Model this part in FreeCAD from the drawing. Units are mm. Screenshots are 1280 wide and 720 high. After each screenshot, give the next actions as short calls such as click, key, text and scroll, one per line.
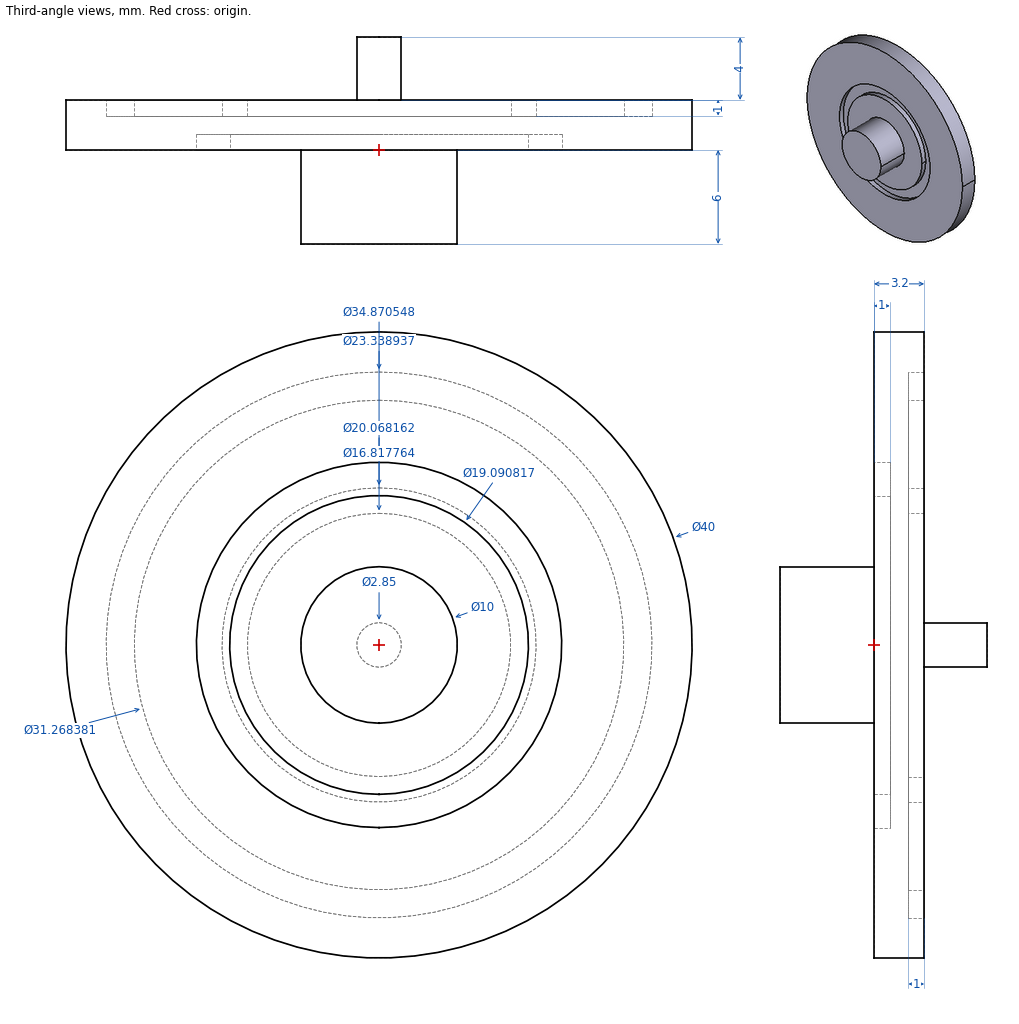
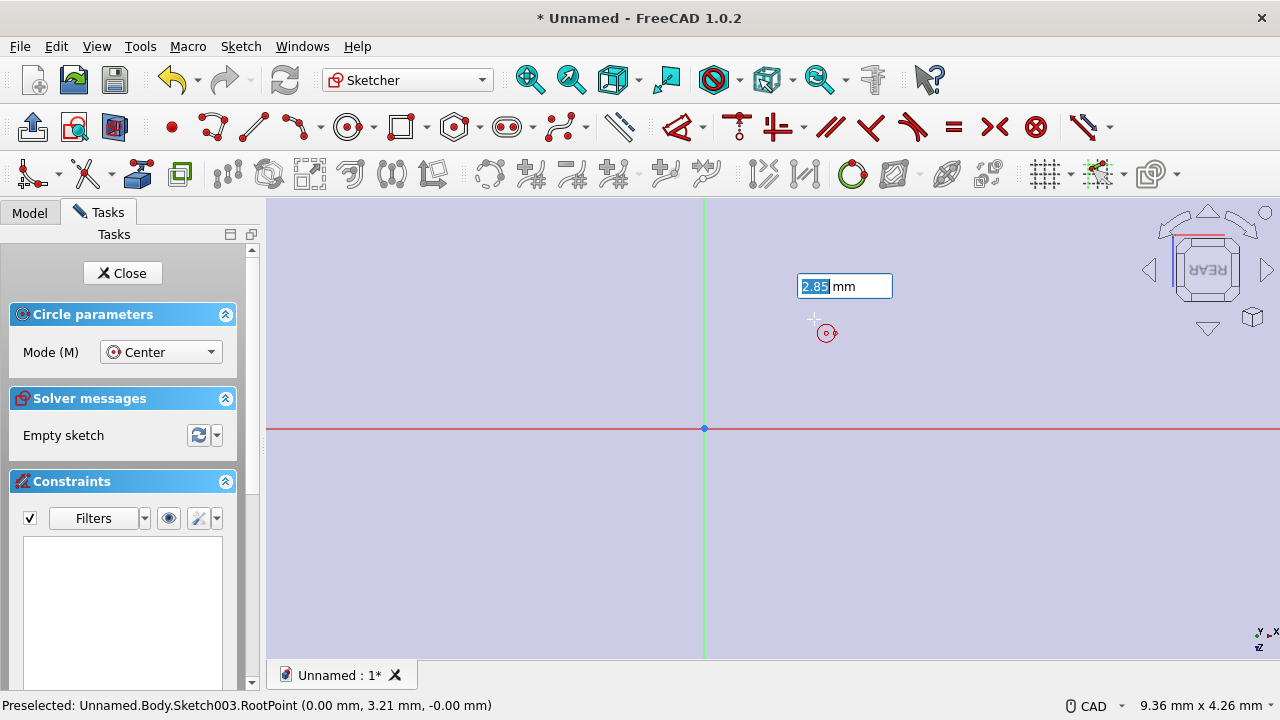
text(2.85)
key(Return)
key(Escape)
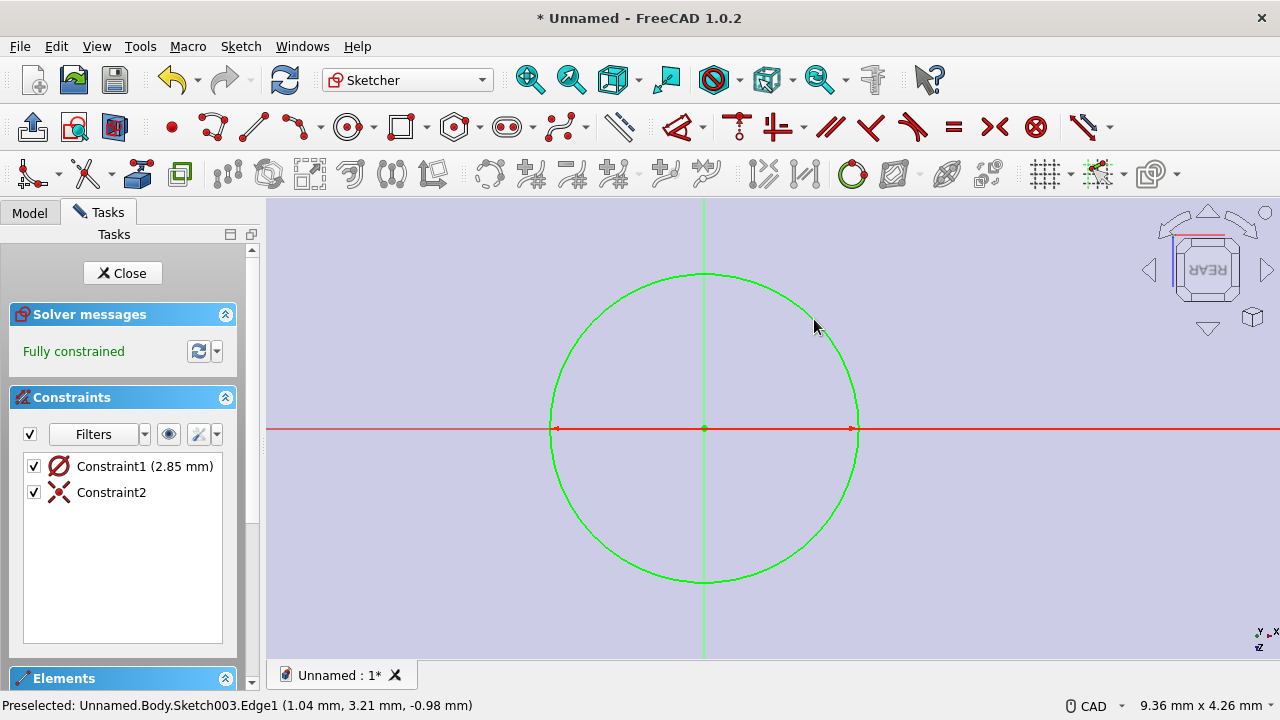
click(123, 273)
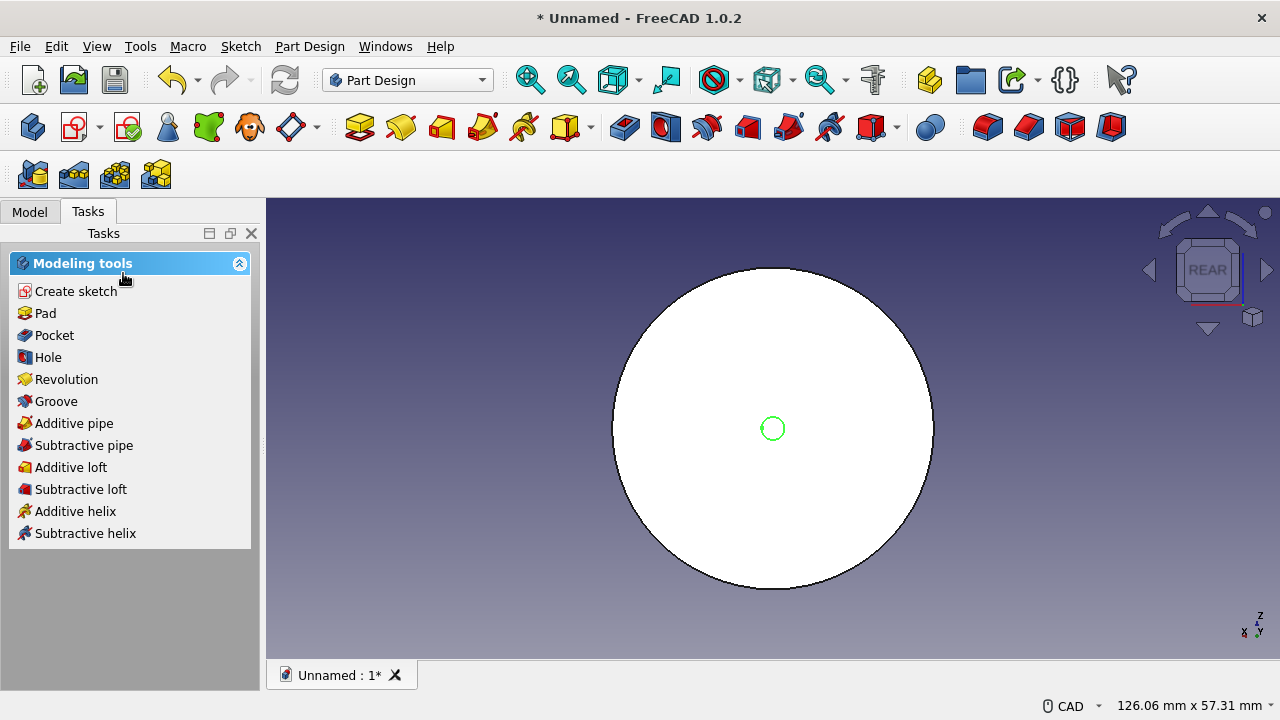
click(360, 128)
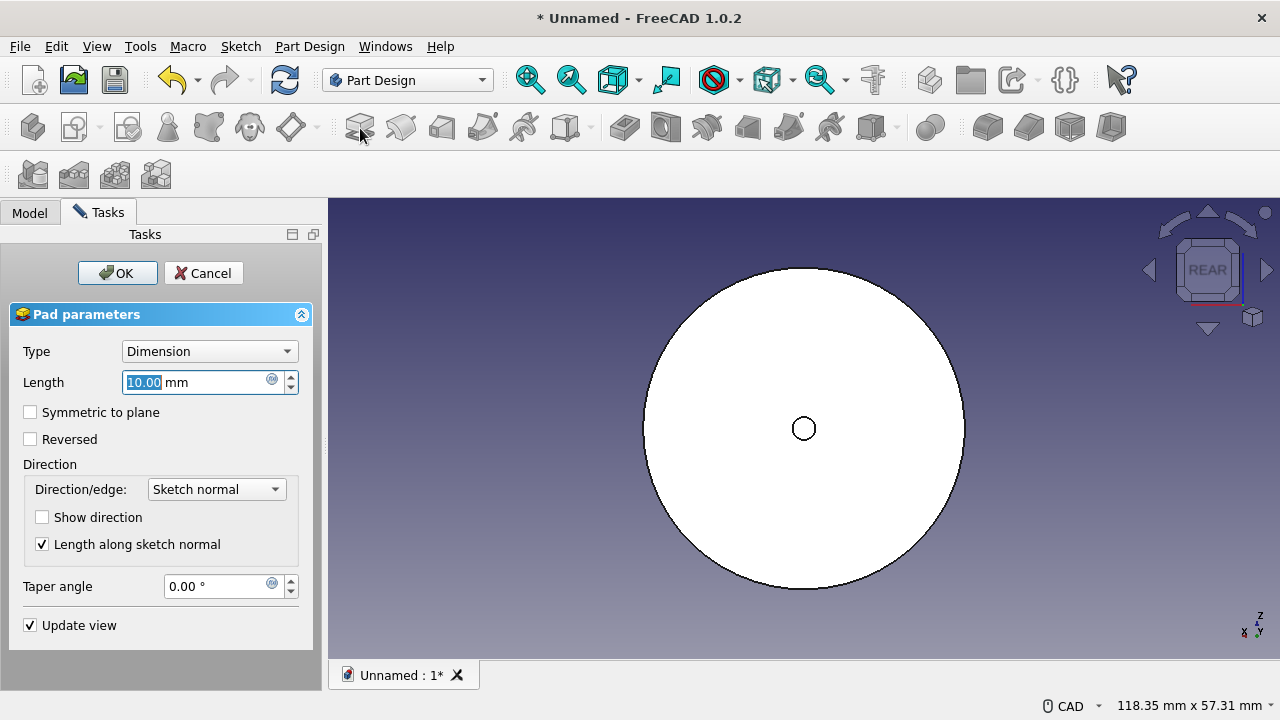
text(4)
key(Tab)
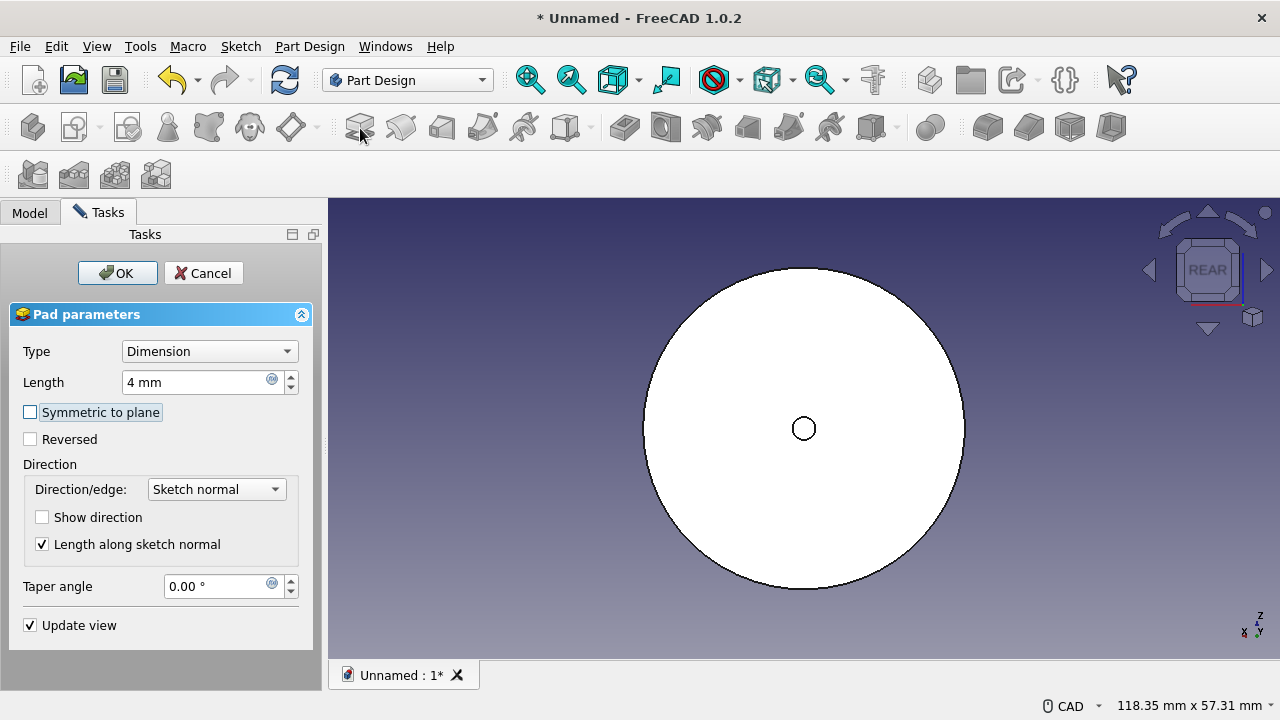
click(118, 273)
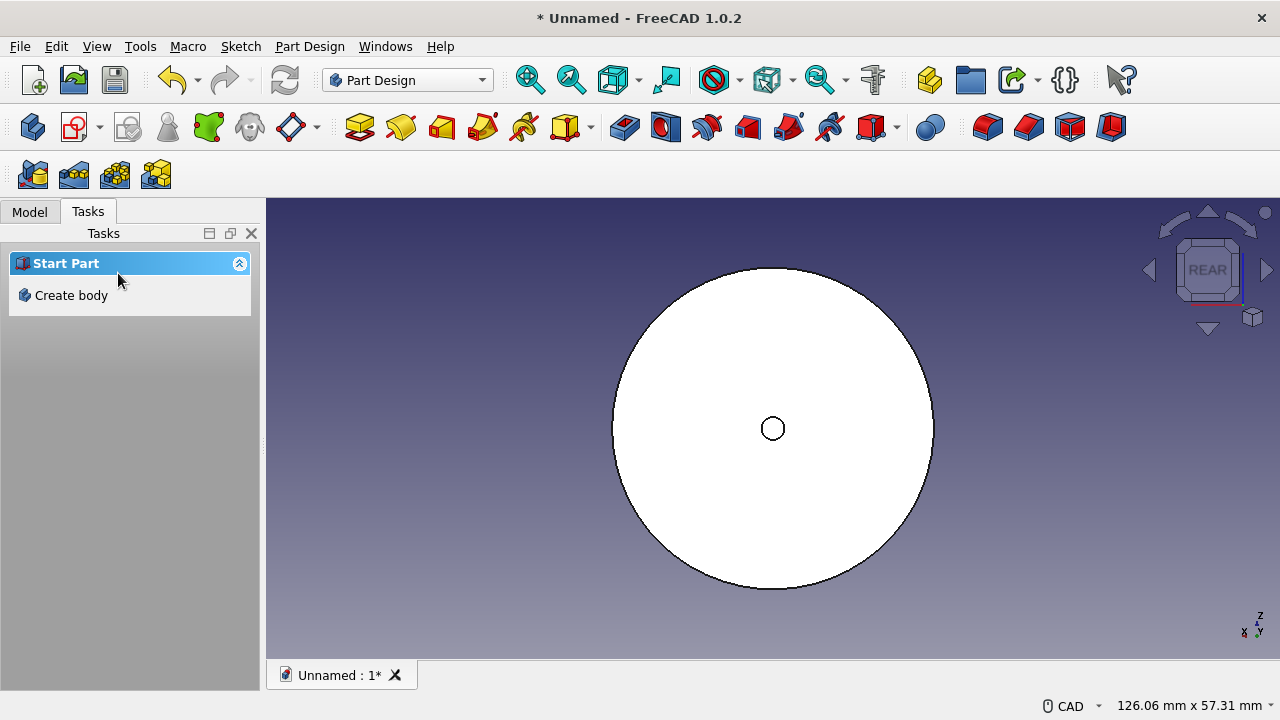
click(681, 428)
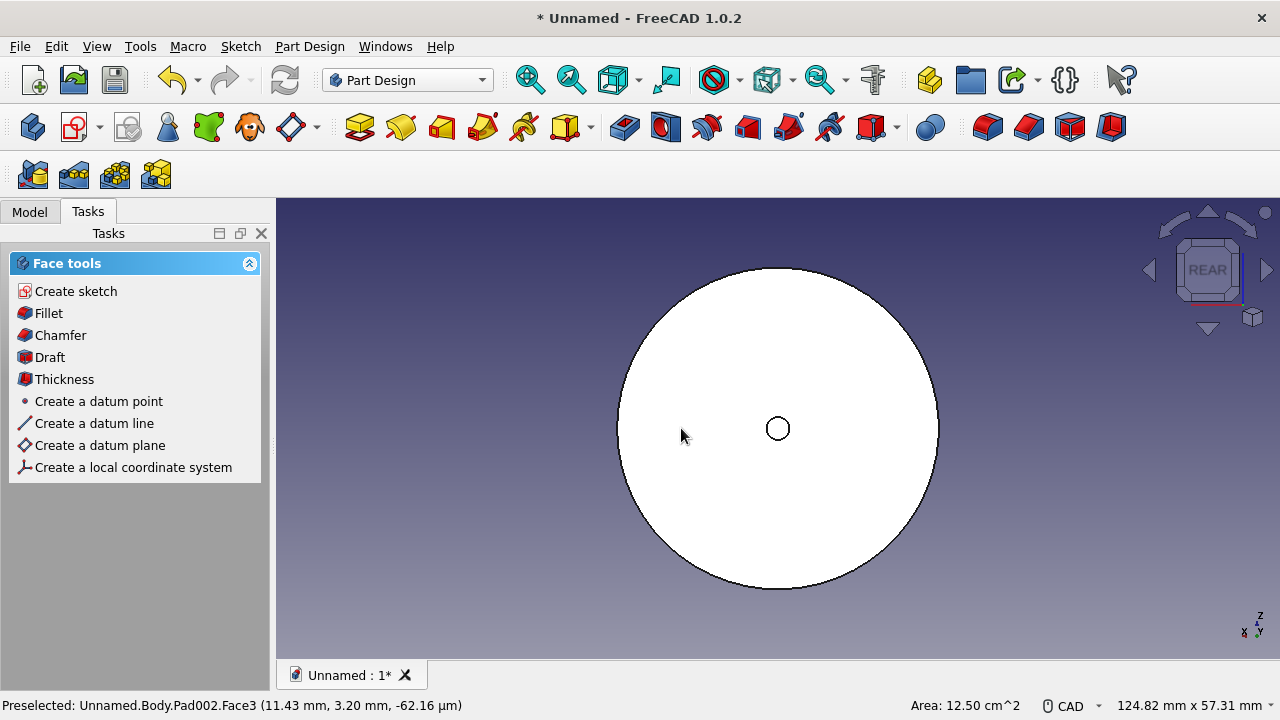
click(74, 128)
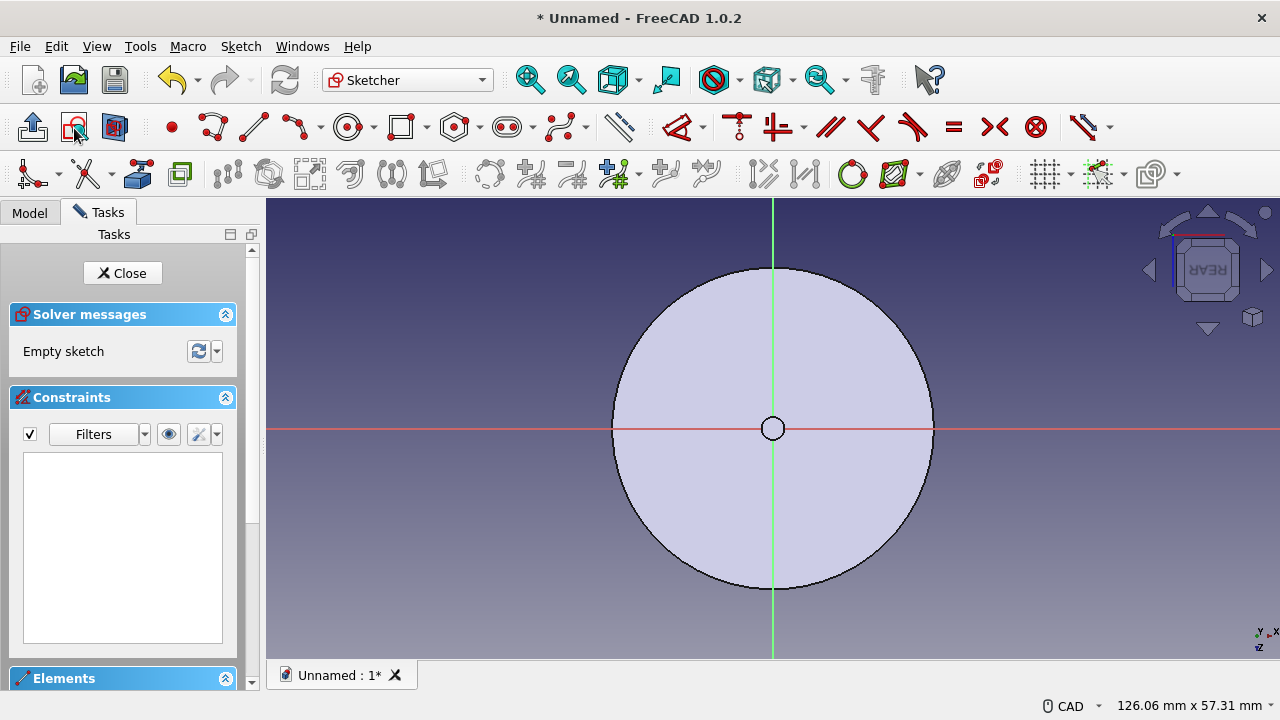
click(348, 128)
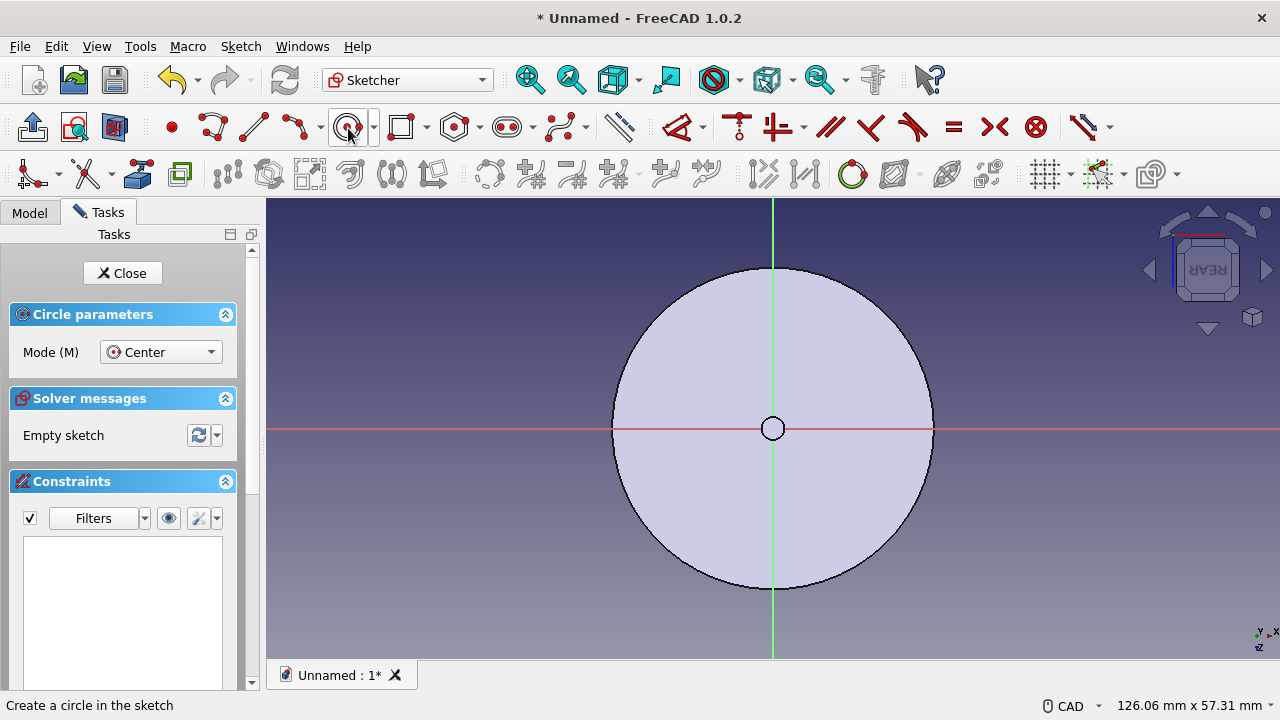
click(773, 428)
move(872, 329)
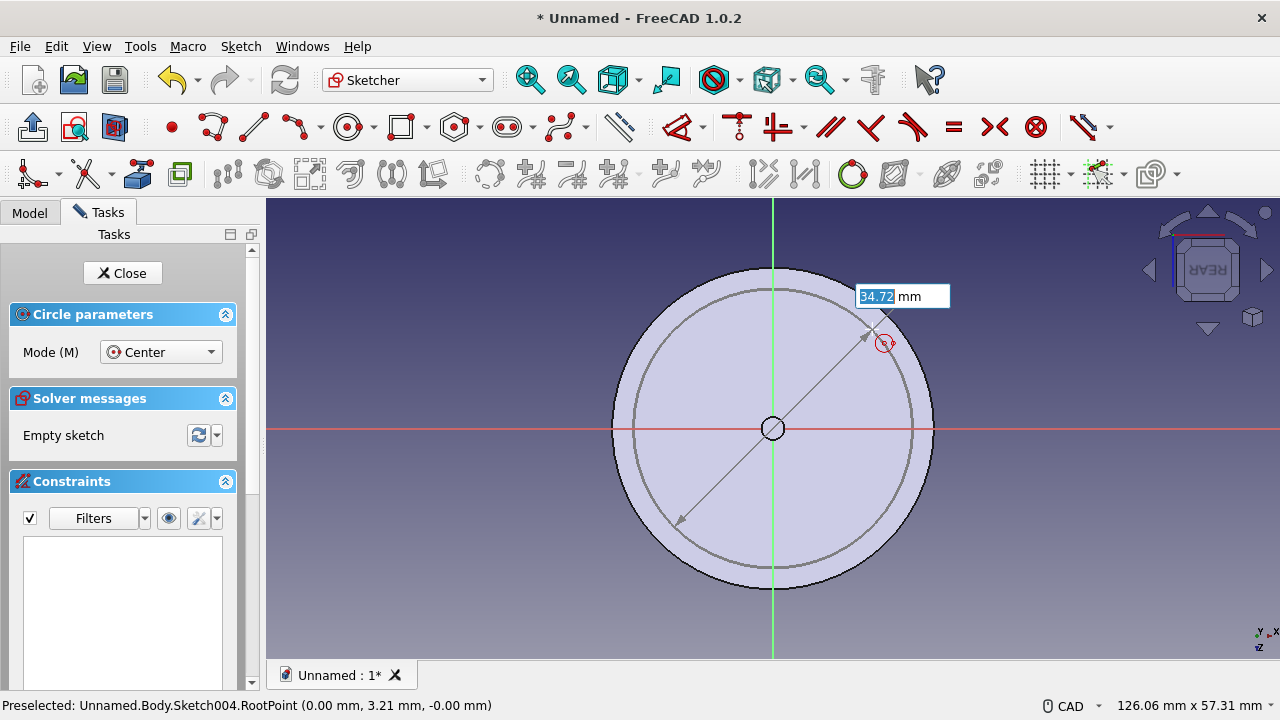
text(34.870548)
key(Return)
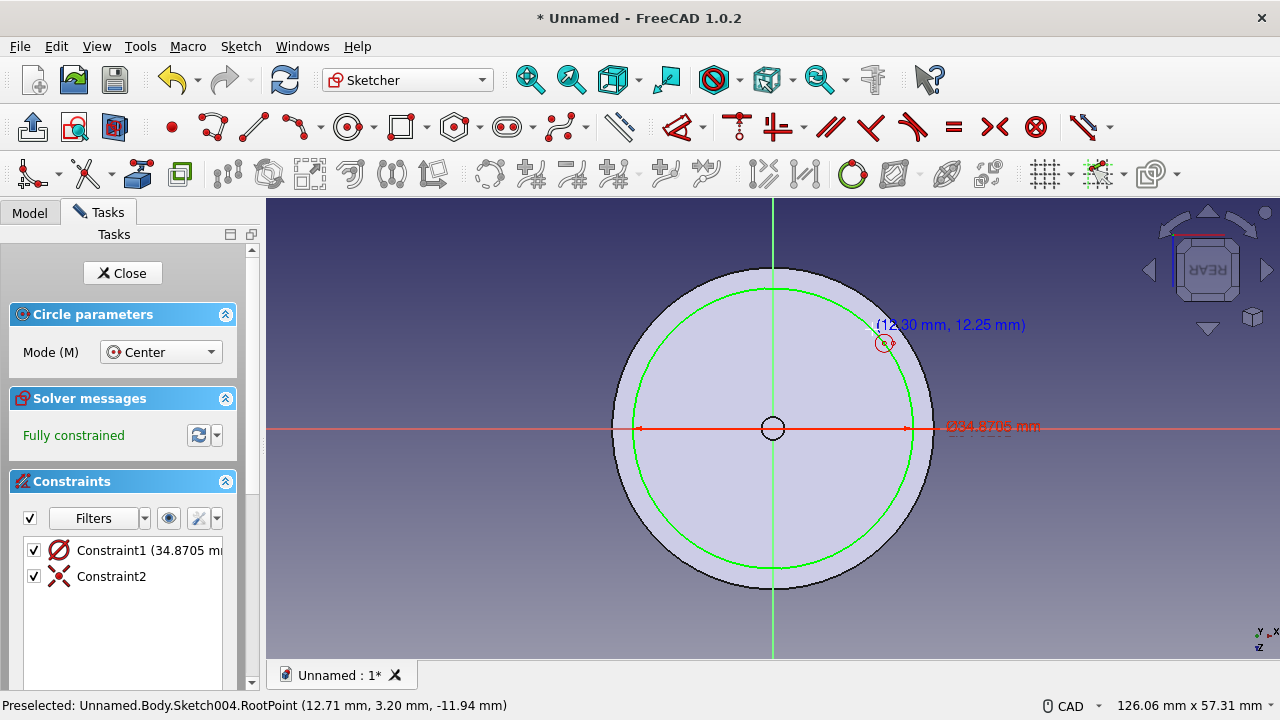
click(773, 428)
move(862, 340)